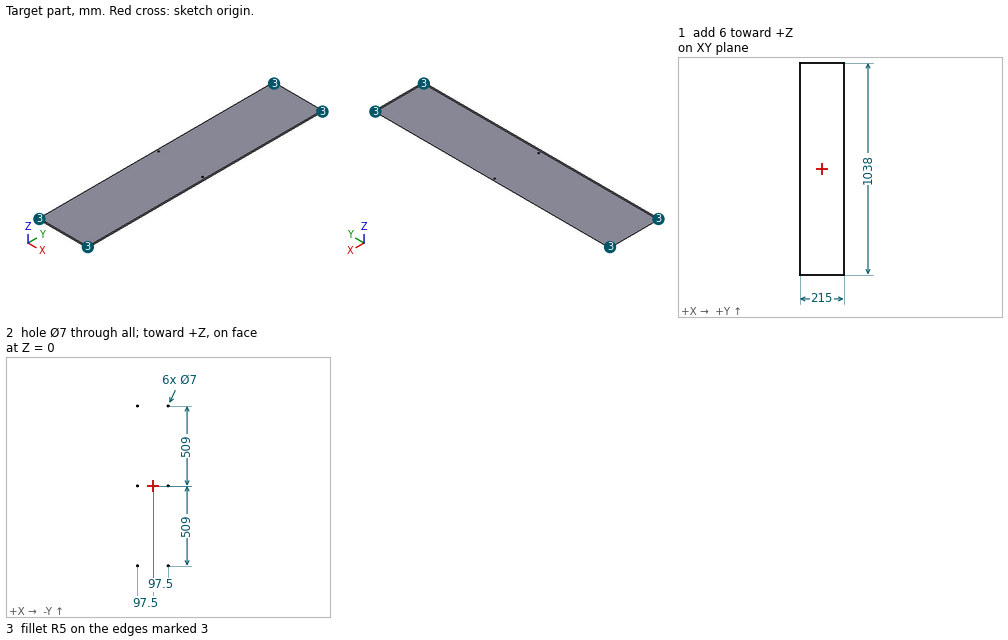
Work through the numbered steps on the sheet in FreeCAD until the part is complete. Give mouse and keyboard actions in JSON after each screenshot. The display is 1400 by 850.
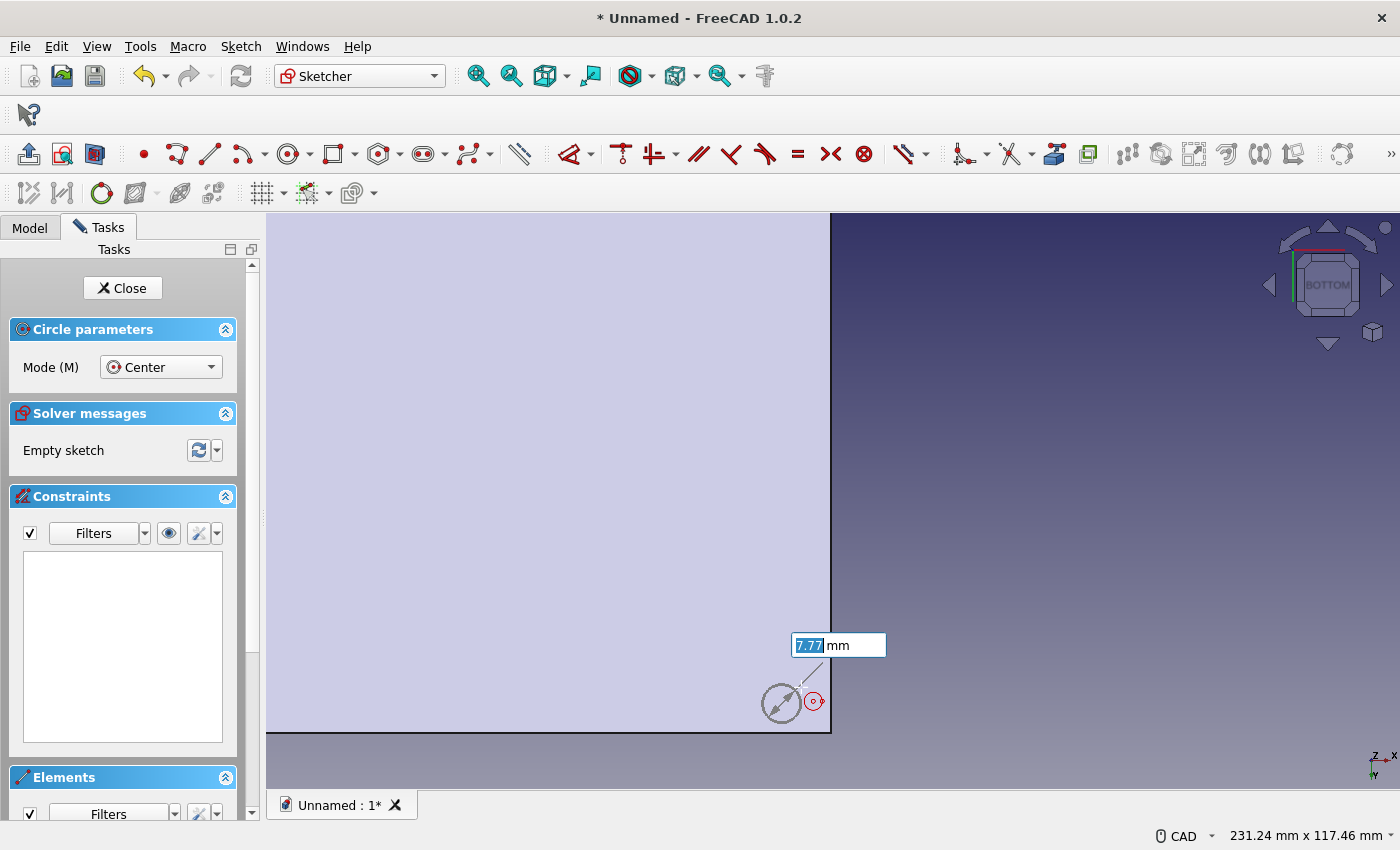
{"action": "left_click", "coordinate": [794, 671]}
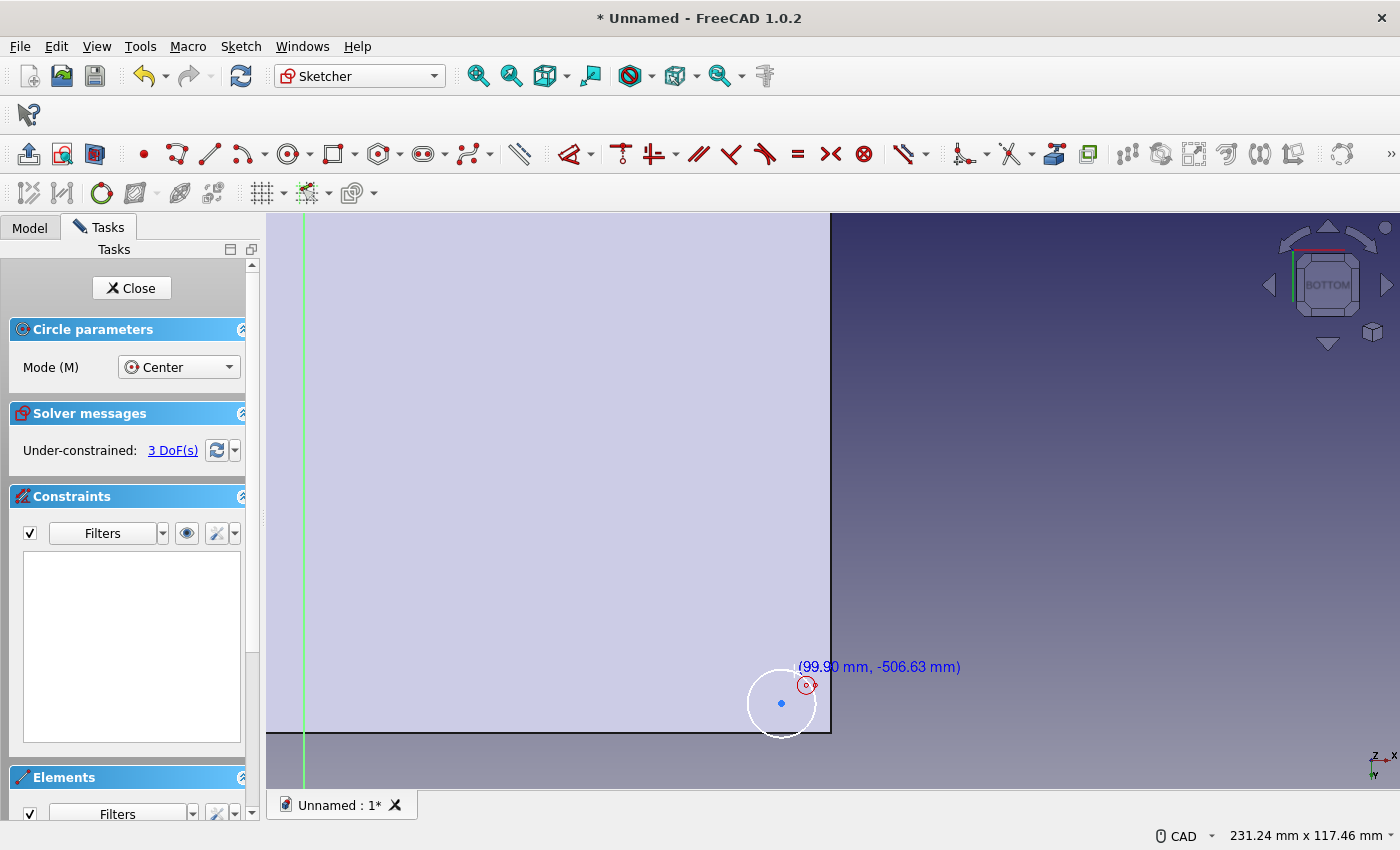
{"action": "scroll", "coordinate": [801, 687], "scroll_direction": "down", "scroll_amount": 13}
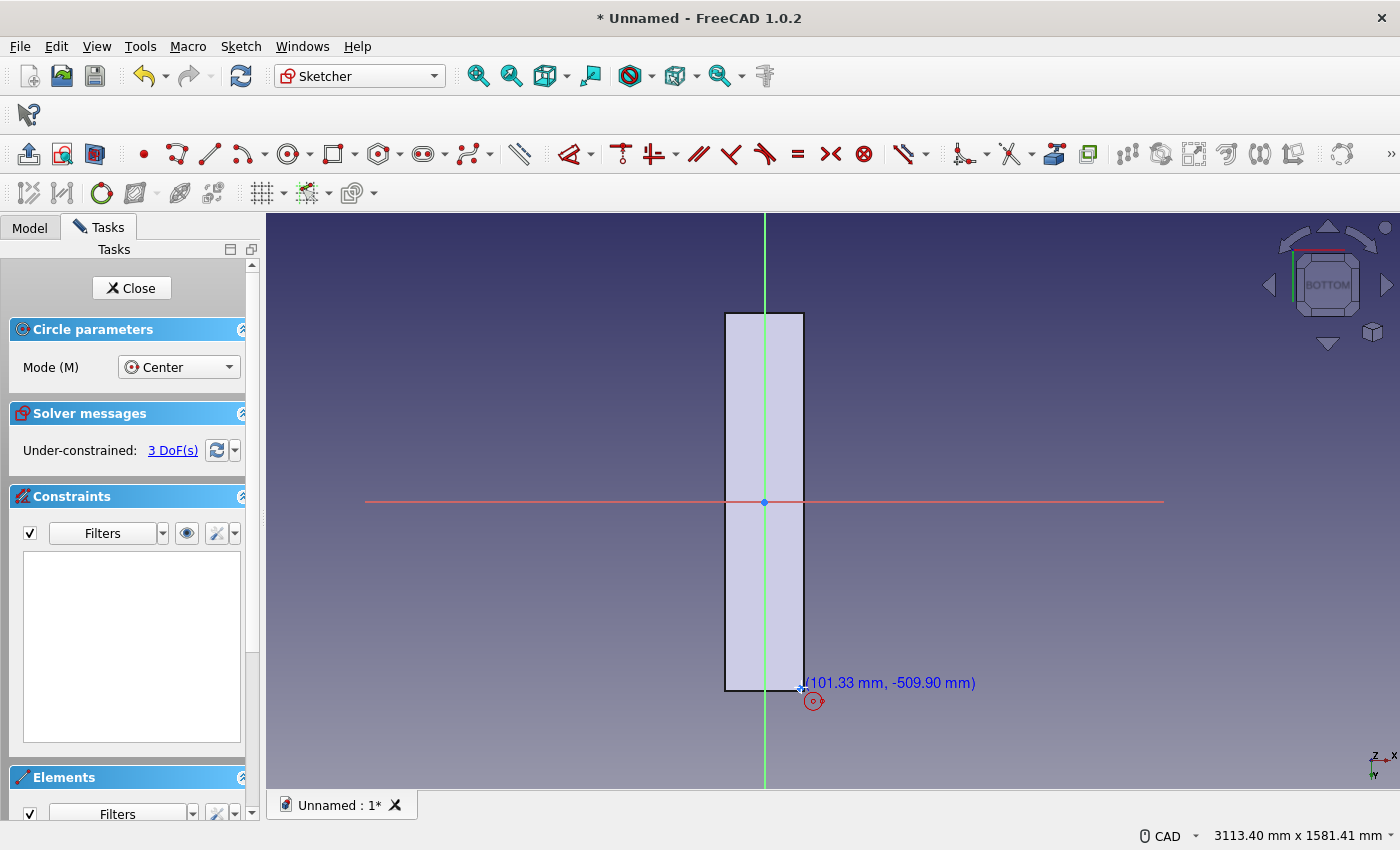
{"action": "scroll", "coordinate": [800, 317], "scroll_direction": "up", "scroll_amount": 15}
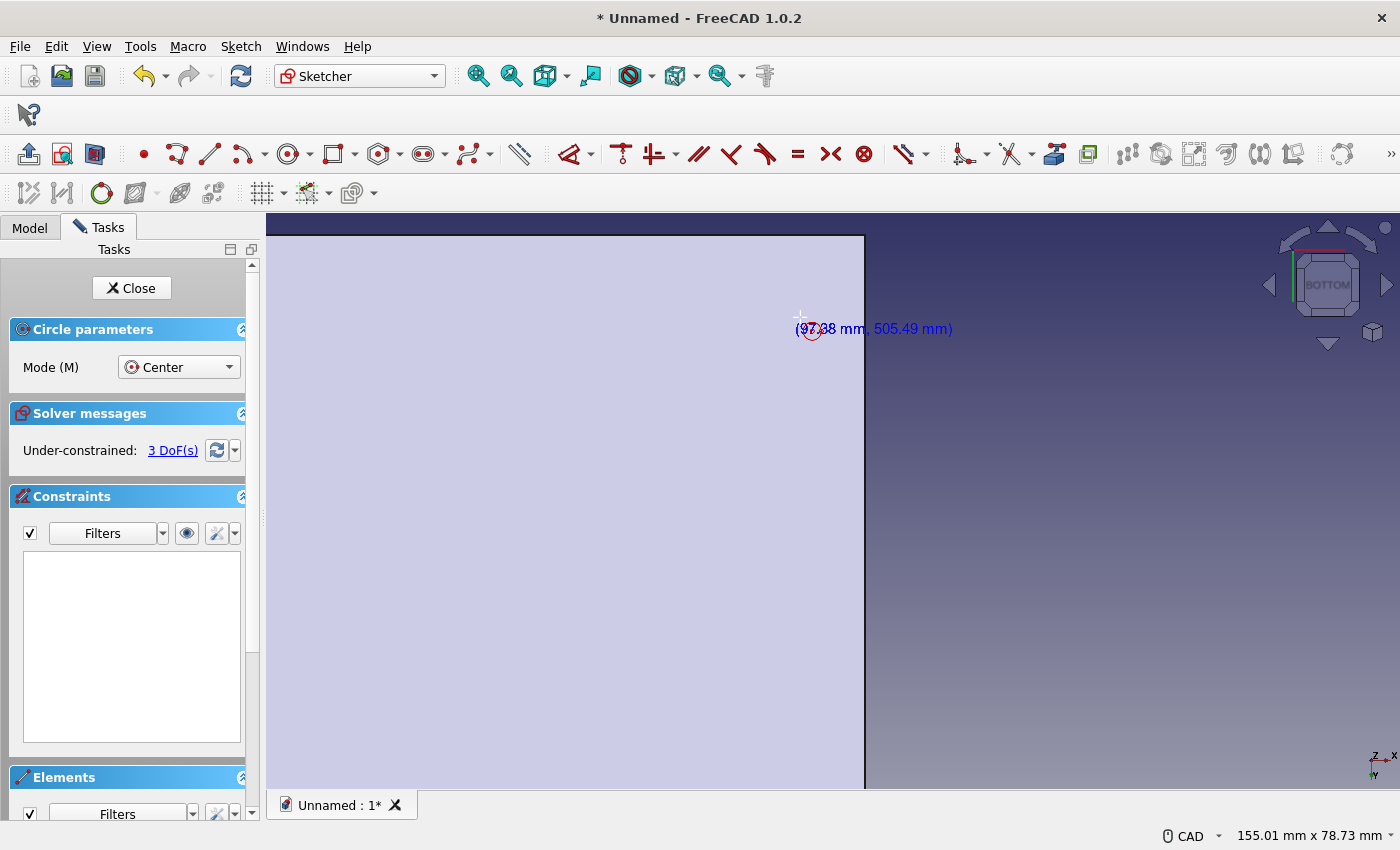
{"action": "scroll", "coordinate": [800, 316], "scroll_direction": "down", "scroll_amount": 15}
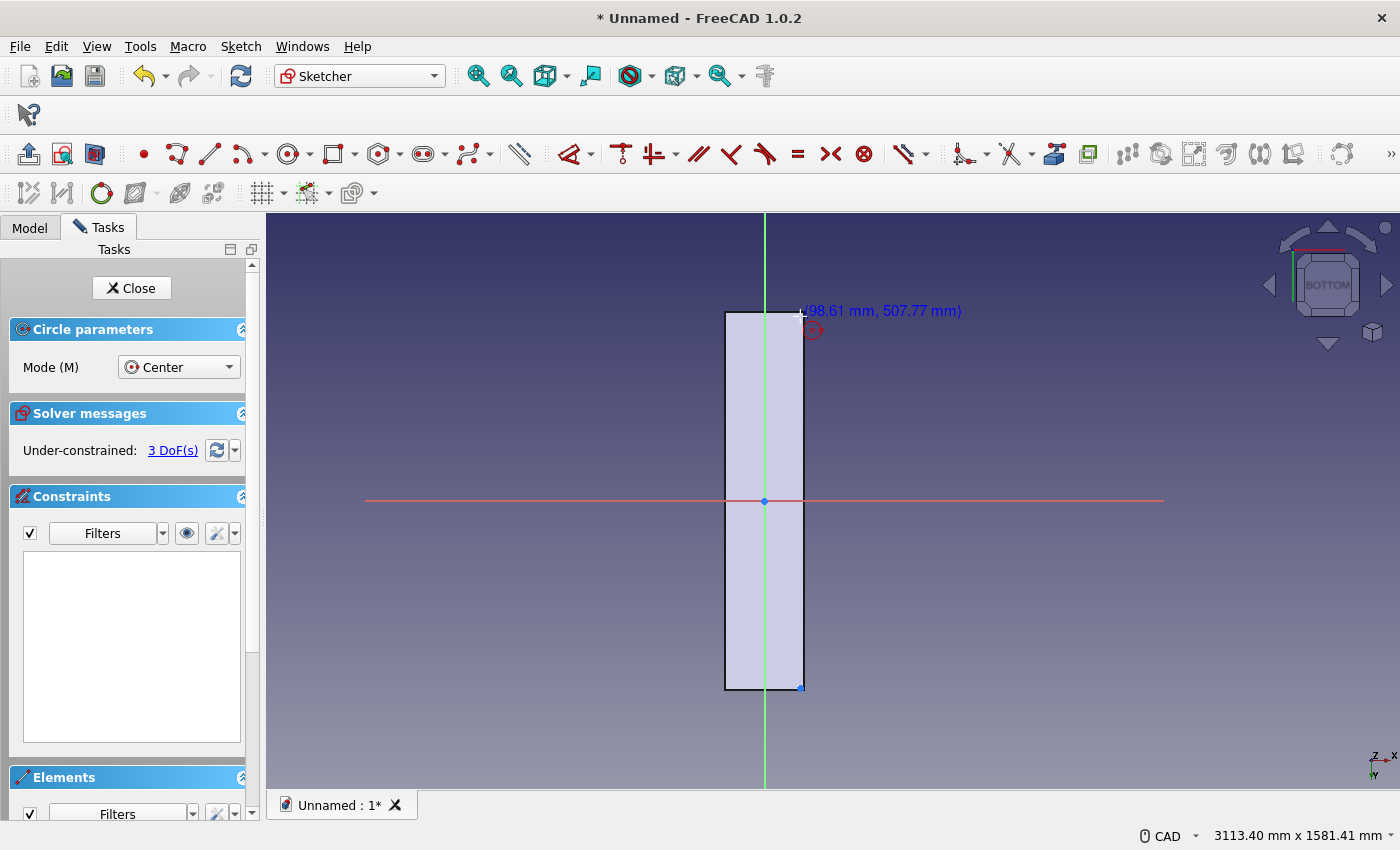
{"action": "left_click", "coordinate": [800, 316]}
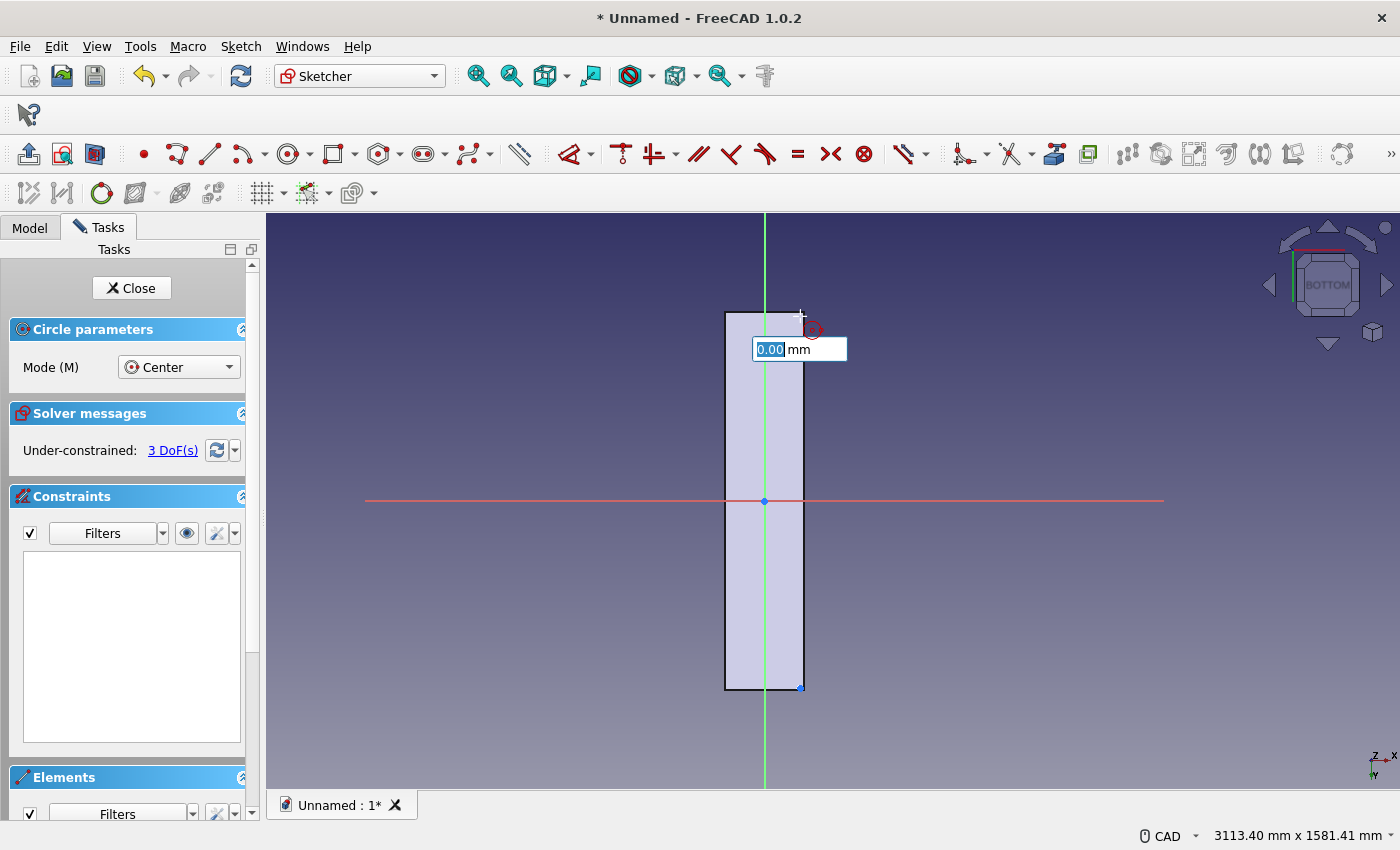
{"action": "scroll", "coordinate": [801, 315], "scroll_direction": "up", "scroll_amount": 13}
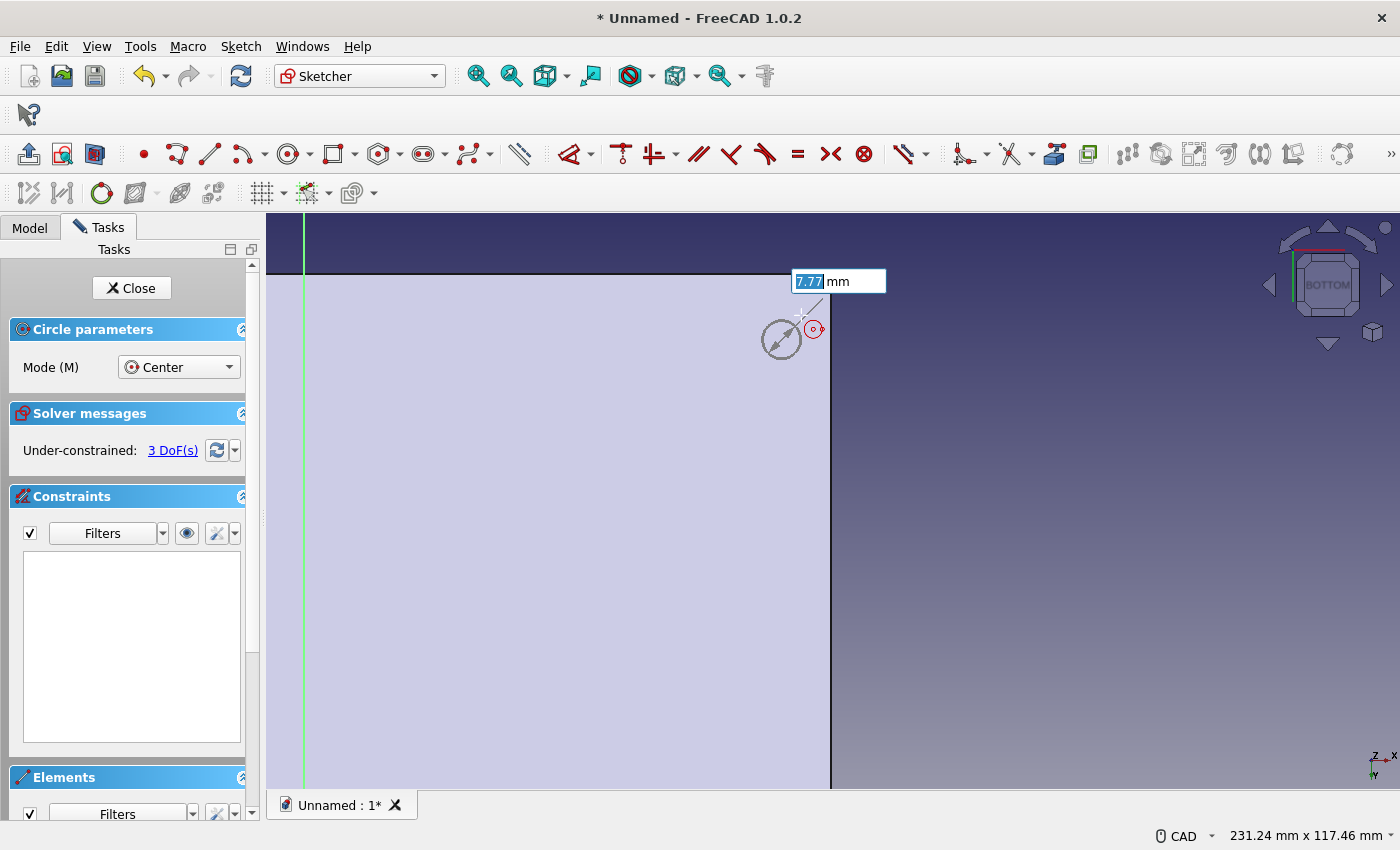
{"action": "left_click", "coordinate": [794, 311]}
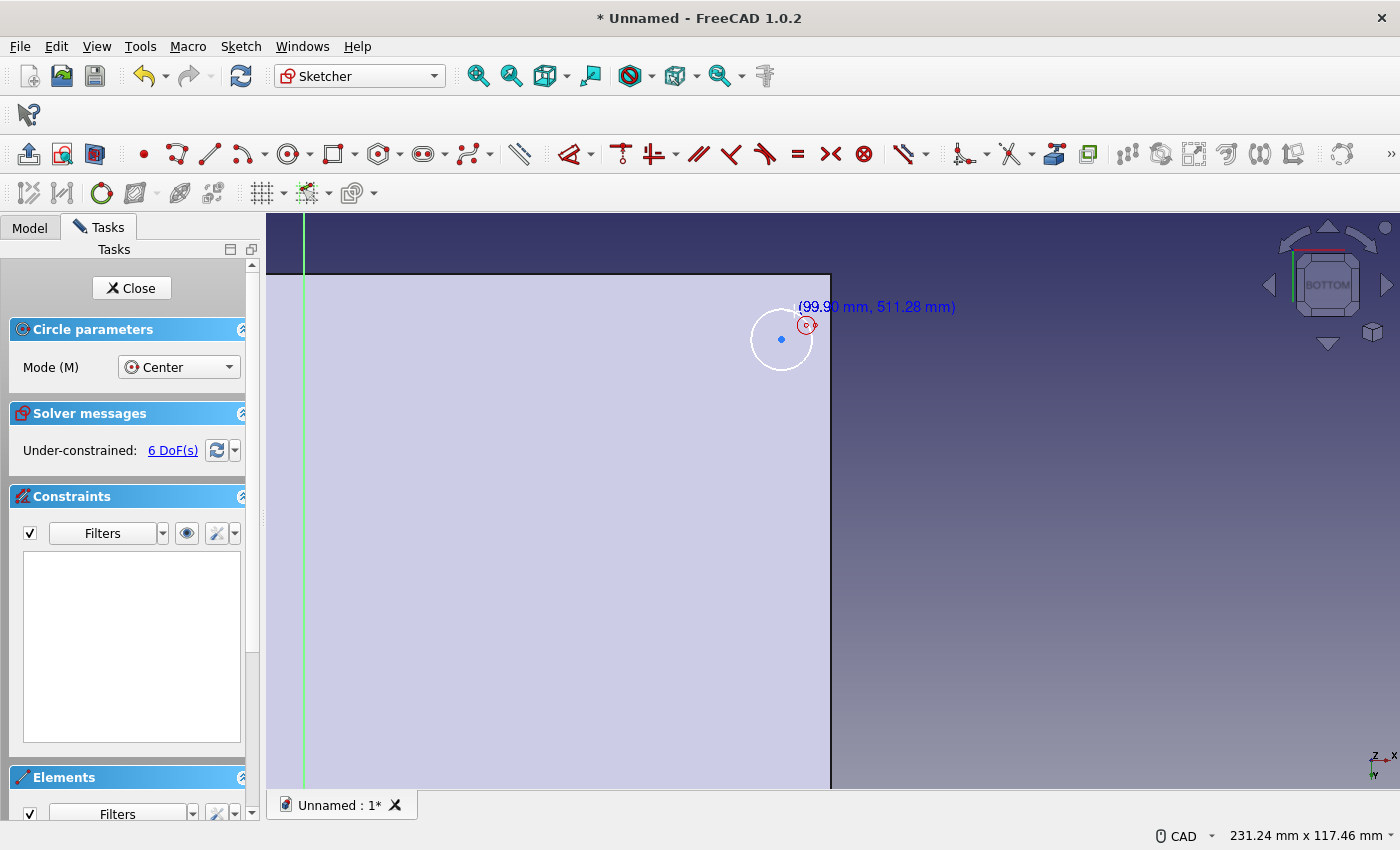
{"action": "scroll", "coordinate": [801, 315], "scroll_direction": "down", "scroll_amount": 13}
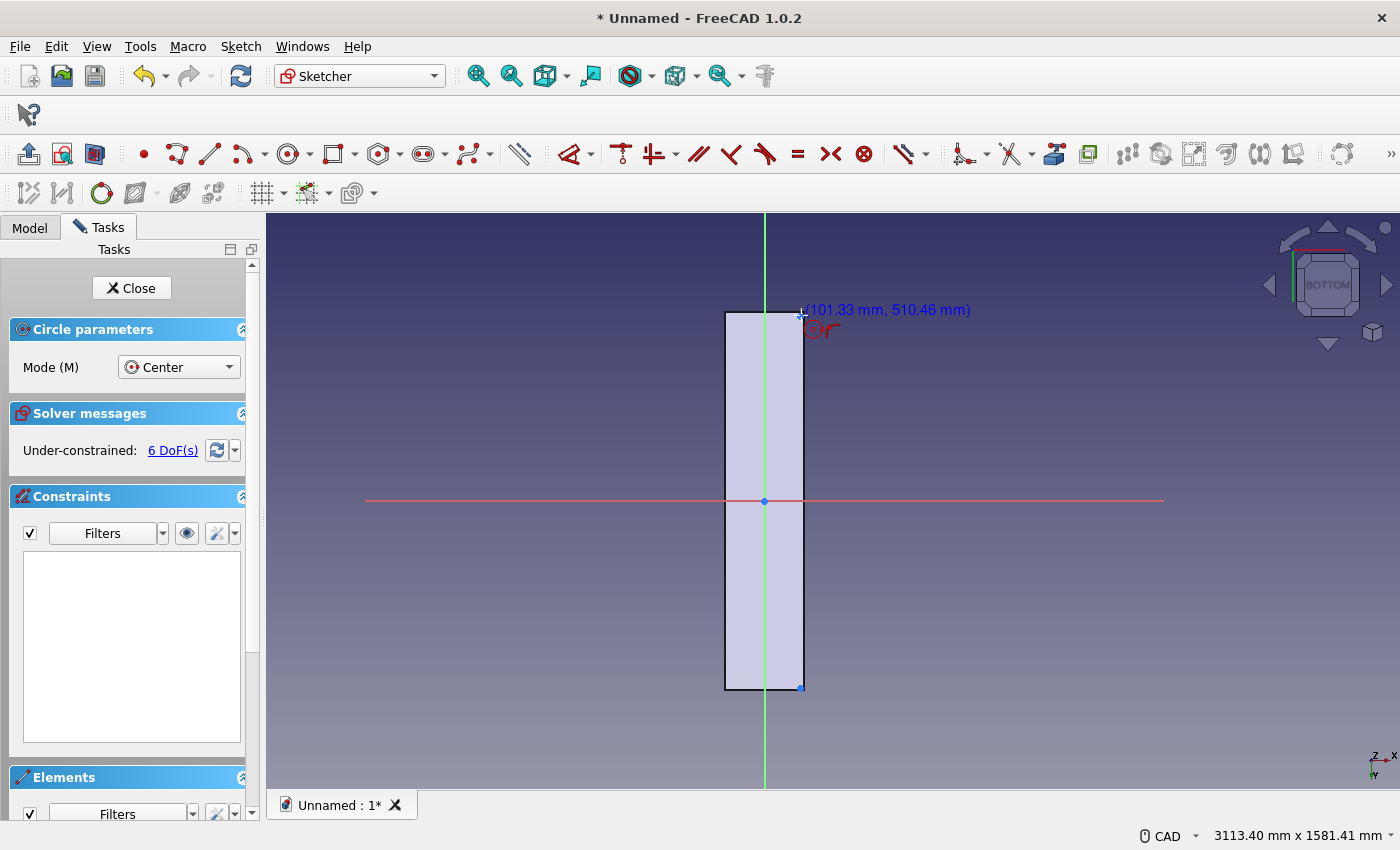
{"action": "scroll", "coordinate": [729, 687], "scroll_direction": "up", "scroll_amount": 15}